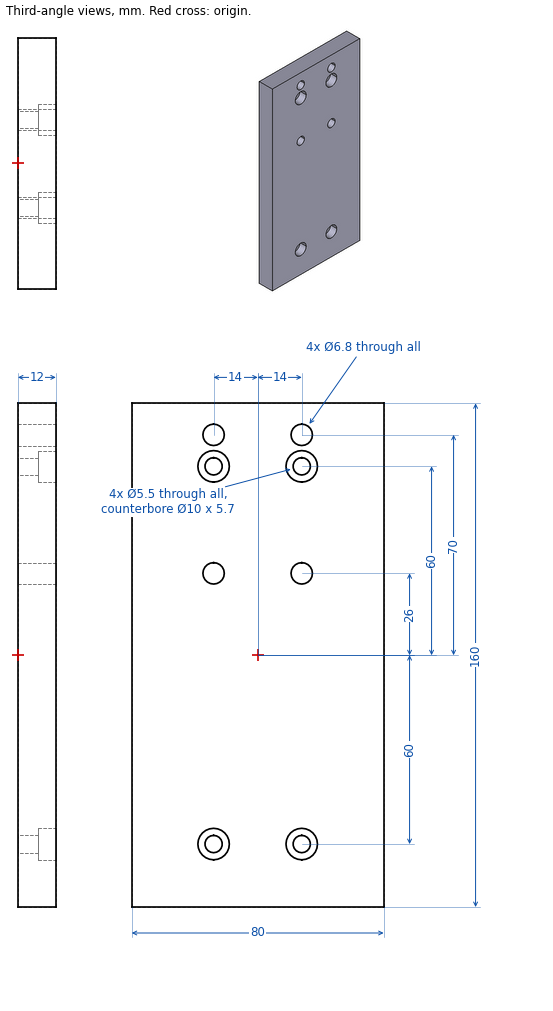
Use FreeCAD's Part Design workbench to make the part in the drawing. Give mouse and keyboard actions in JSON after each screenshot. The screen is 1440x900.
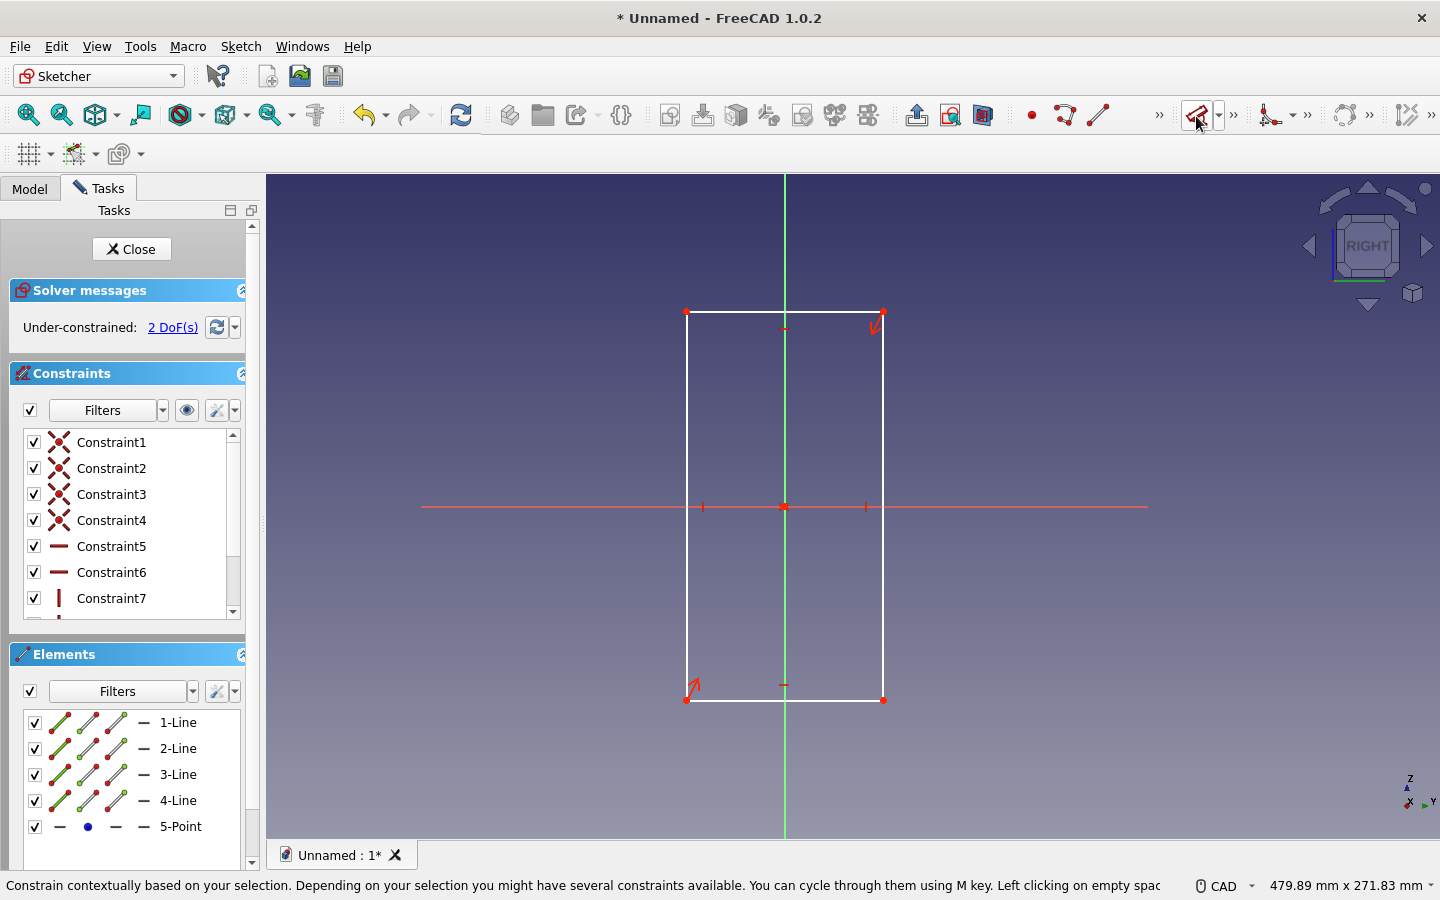
{"action": "left_click", "coordinate": [746, 701]}
{"action": "left_click", "coordinate": [740, 735]}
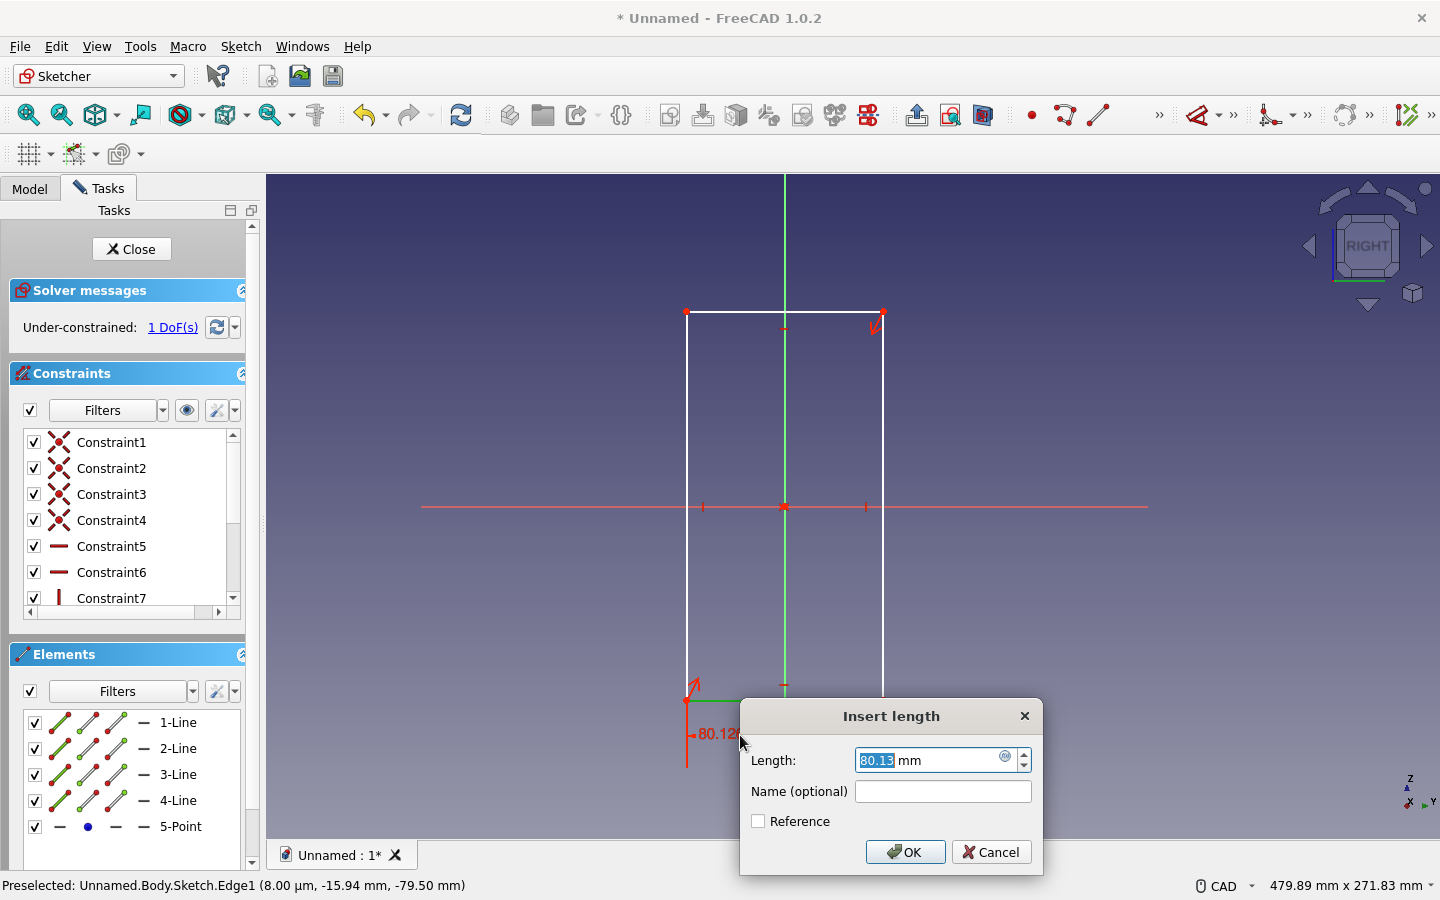
{"action": "type", "text": "80"}
{"action": "key", "text": "Return"}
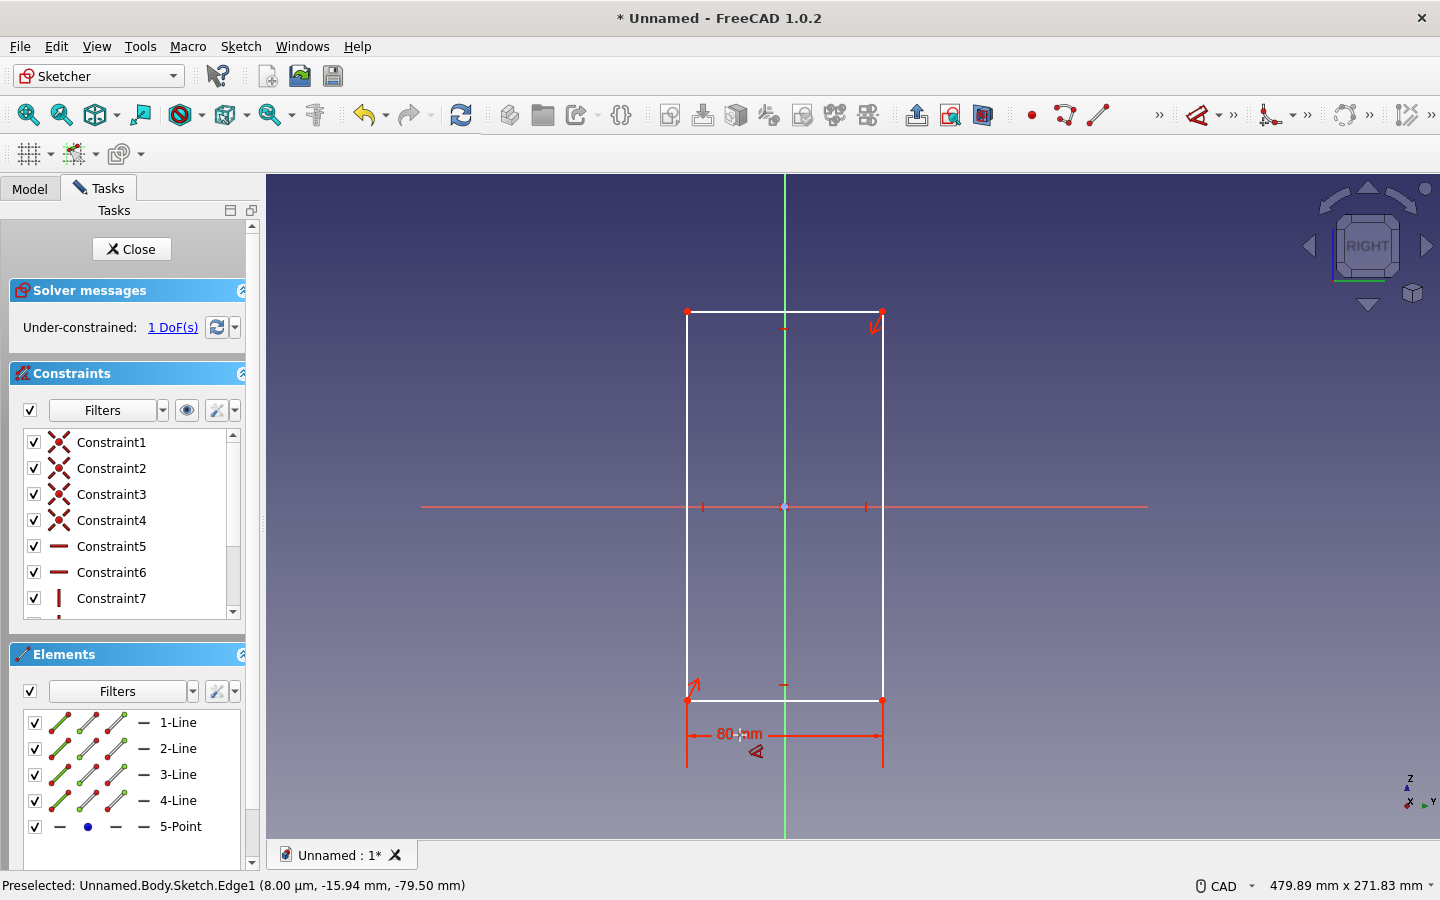
{"action": "left_click", "coordinate": [883, 584]}
{"action": "left_click", "coordinate": [917, 417]}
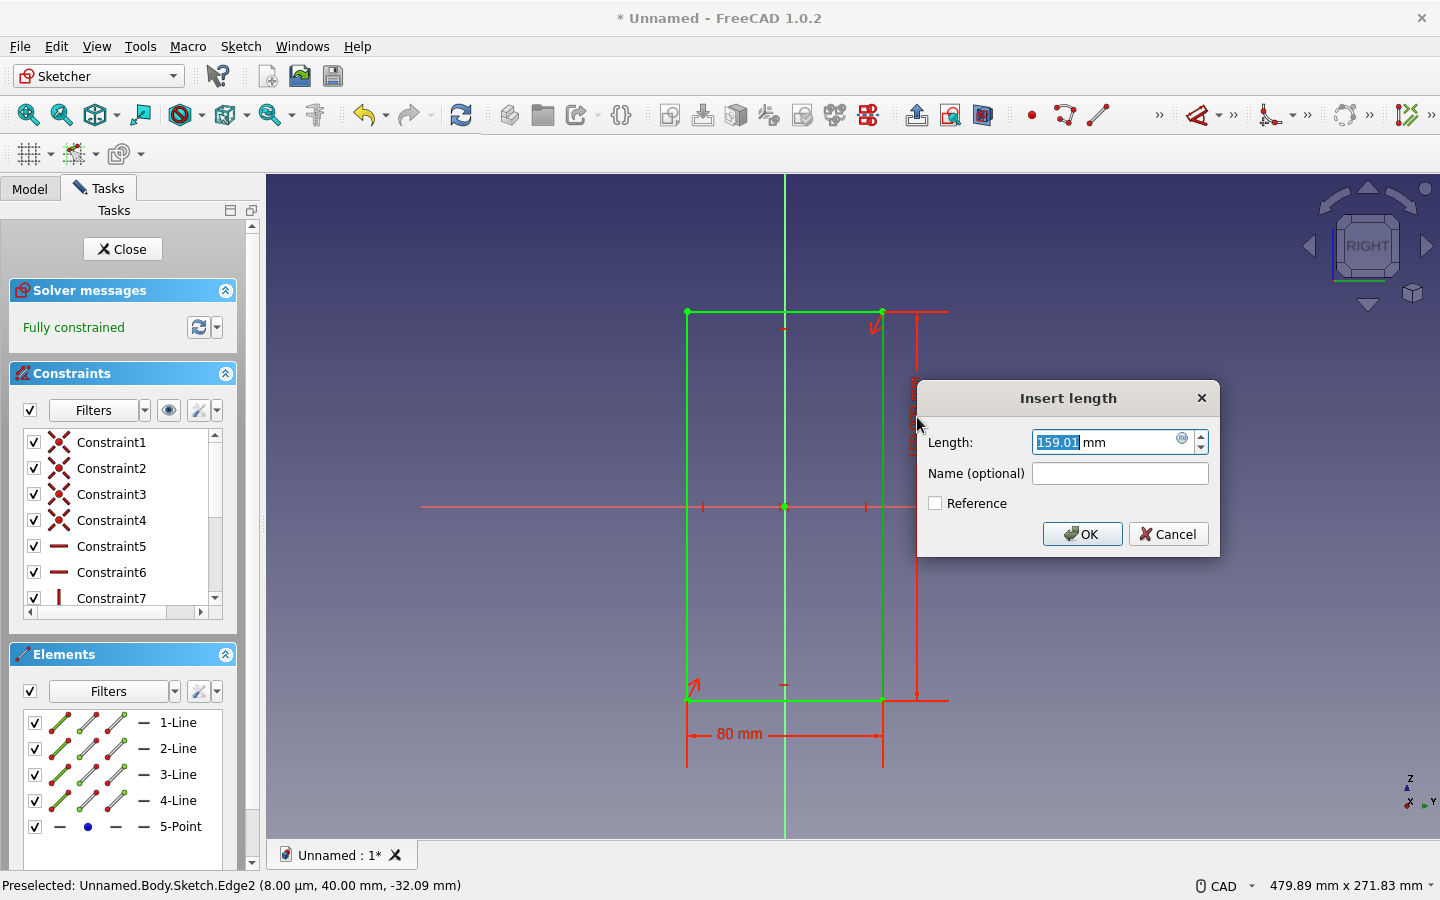
{"action": "type", "text": "160"}
{"action": "key", "text": "Return"}
{"action": "key", "text": "Escape"}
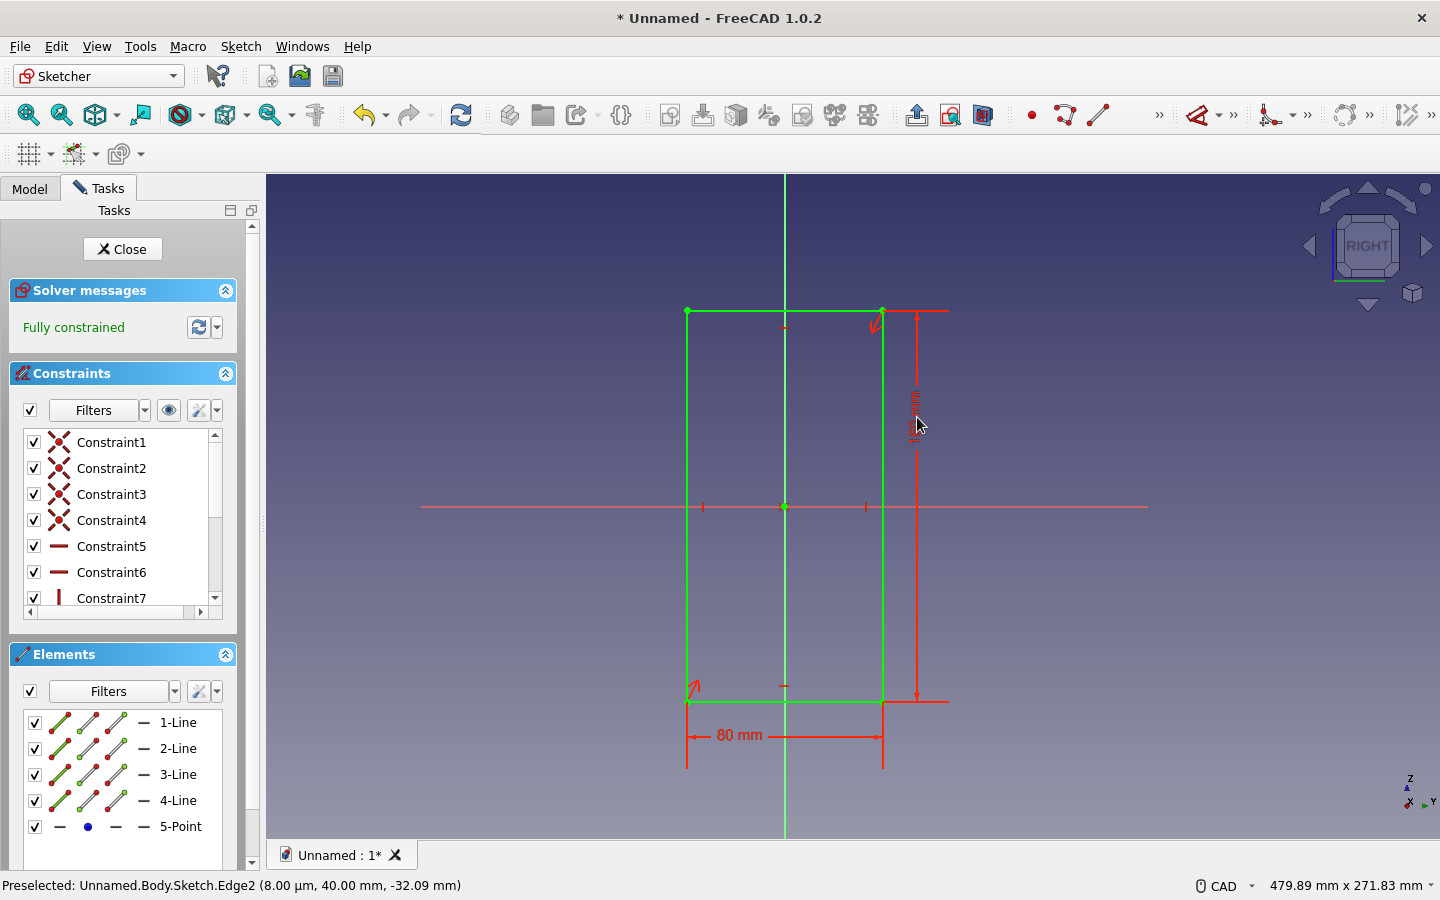
{"action": "left_click", "coordinate": [123, 249]}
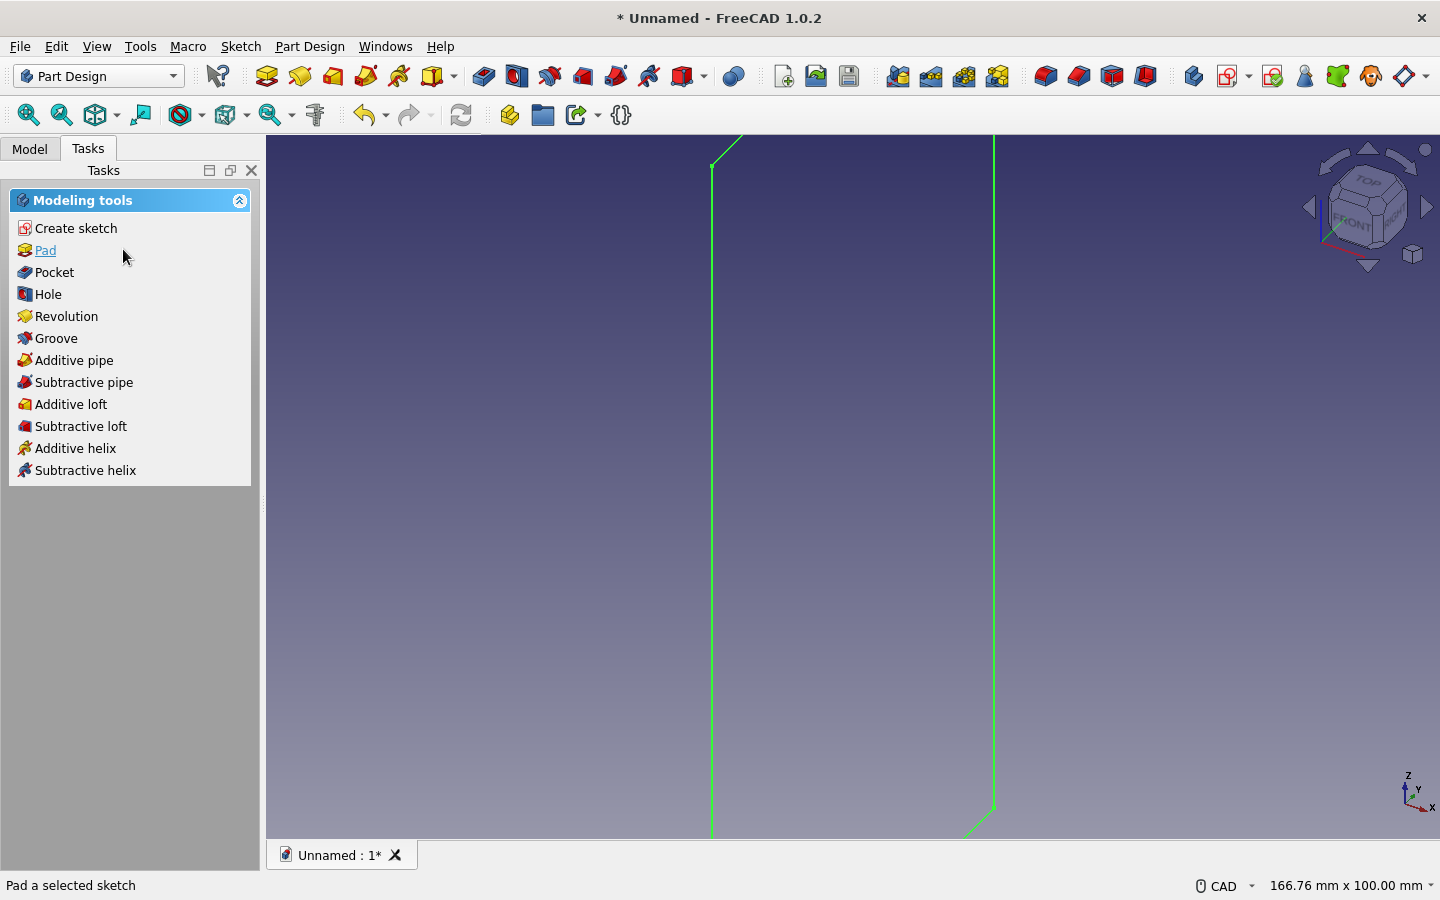
{"action": "left_click", "coordinate": [267, 76]}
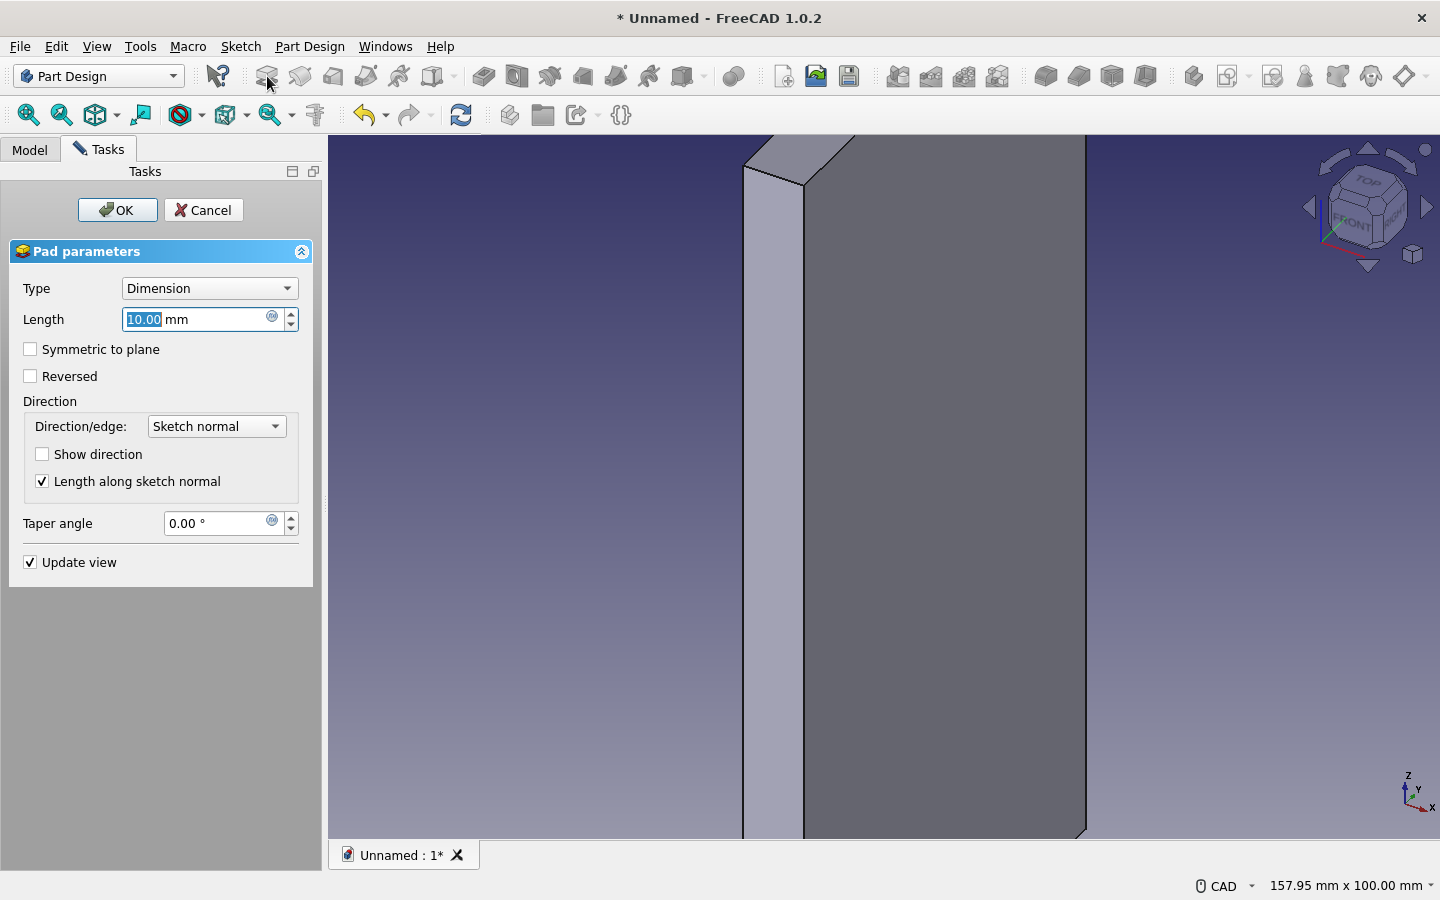
{"action": "type", "text": "12"}
{"action": "key", "text": "Tab"}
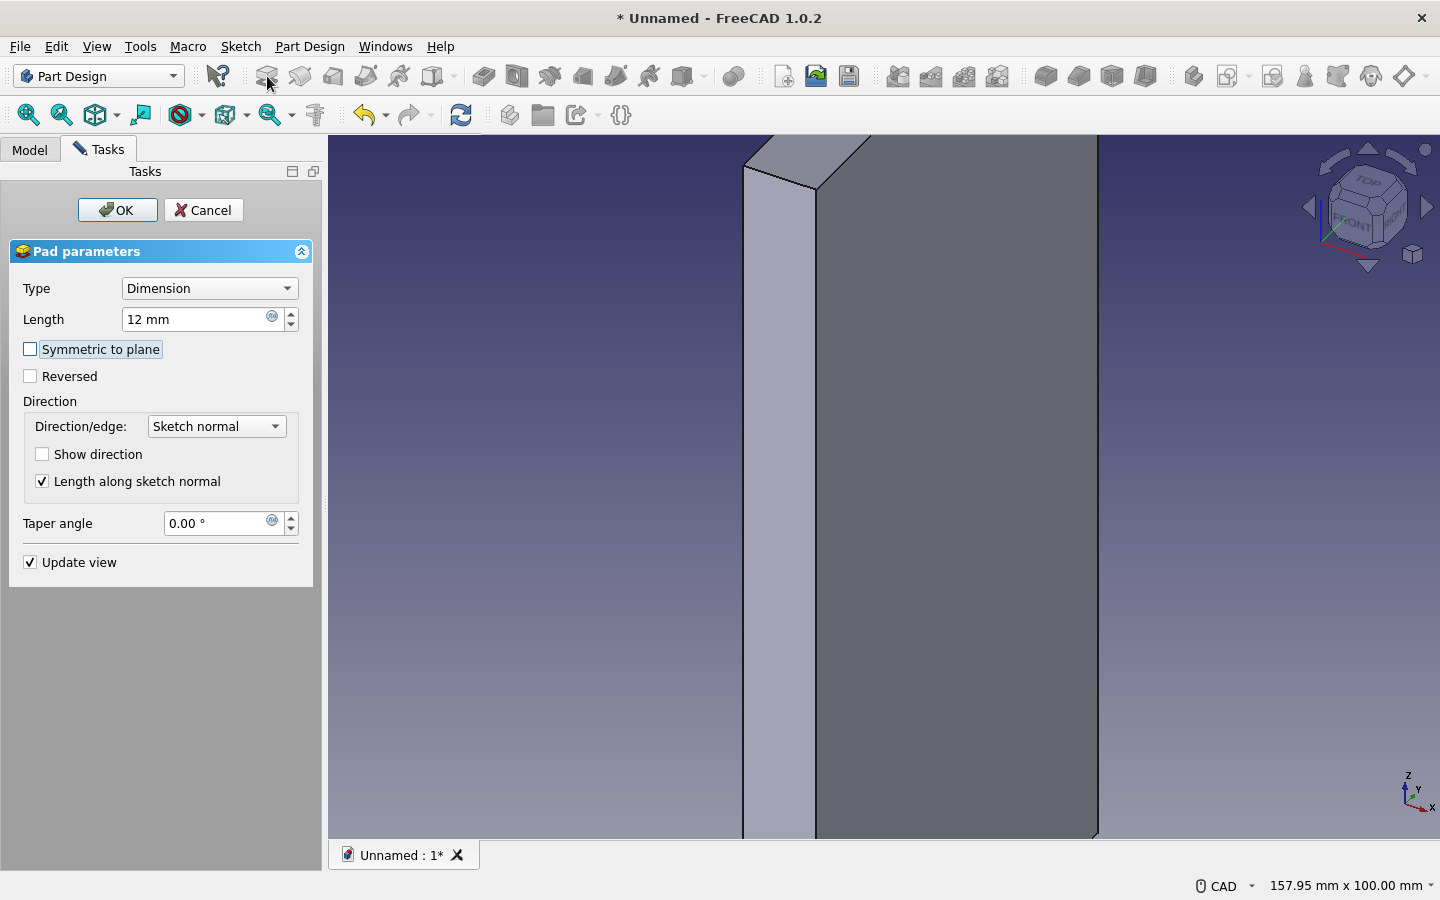
{"action": "left_click", "coordinate": [118, 210]}